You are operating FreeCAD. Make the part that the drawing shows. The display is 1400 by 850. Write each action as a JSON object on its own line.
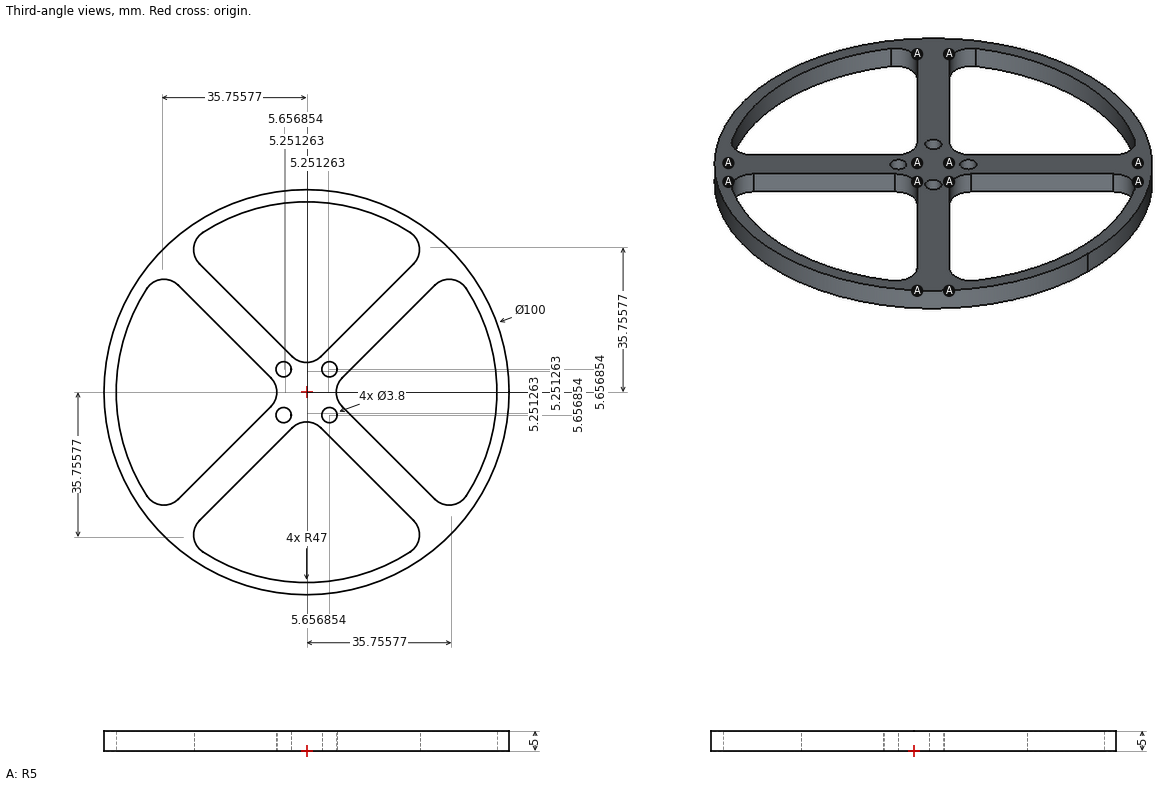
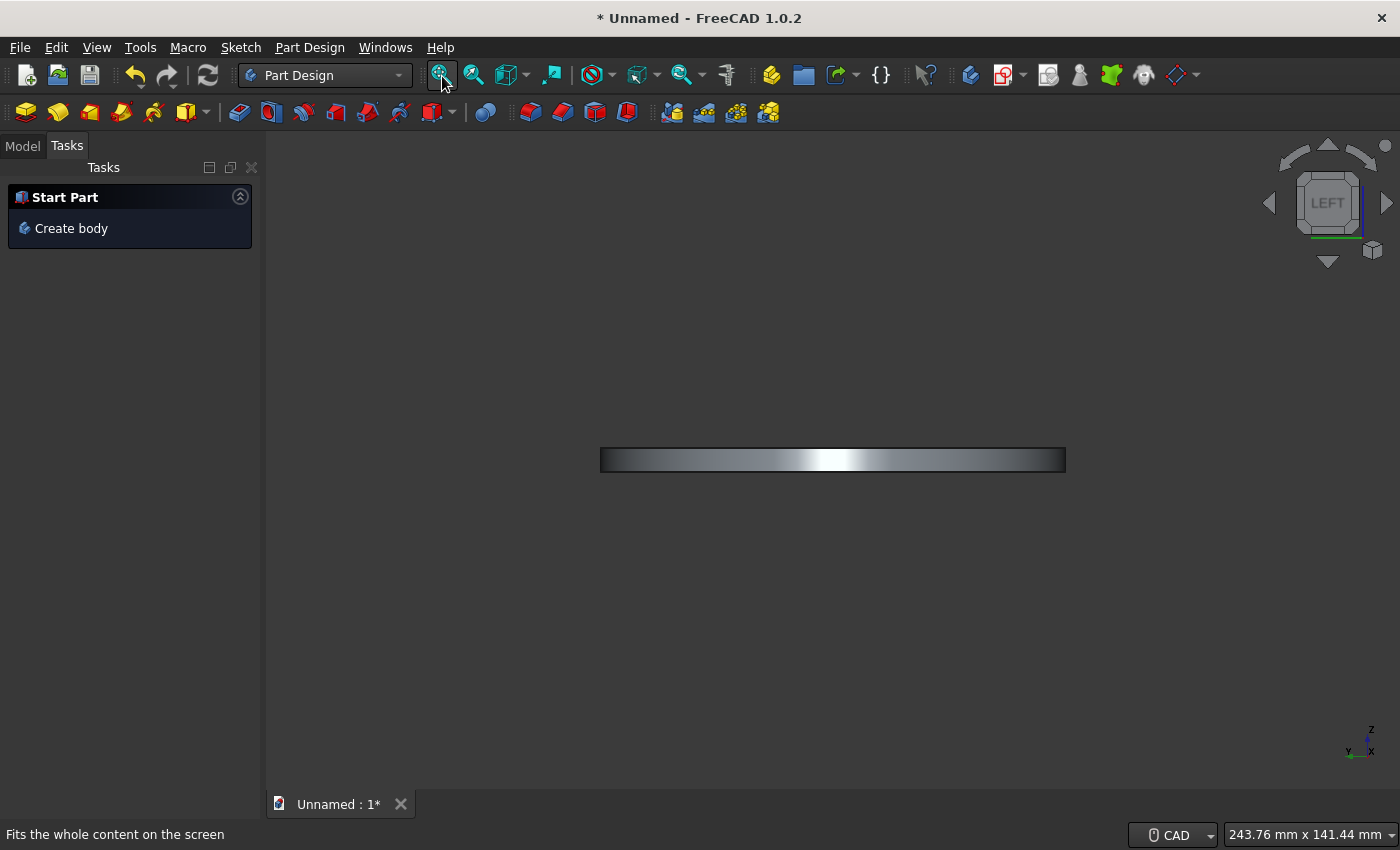
{"action": "key", "text": "v 3"}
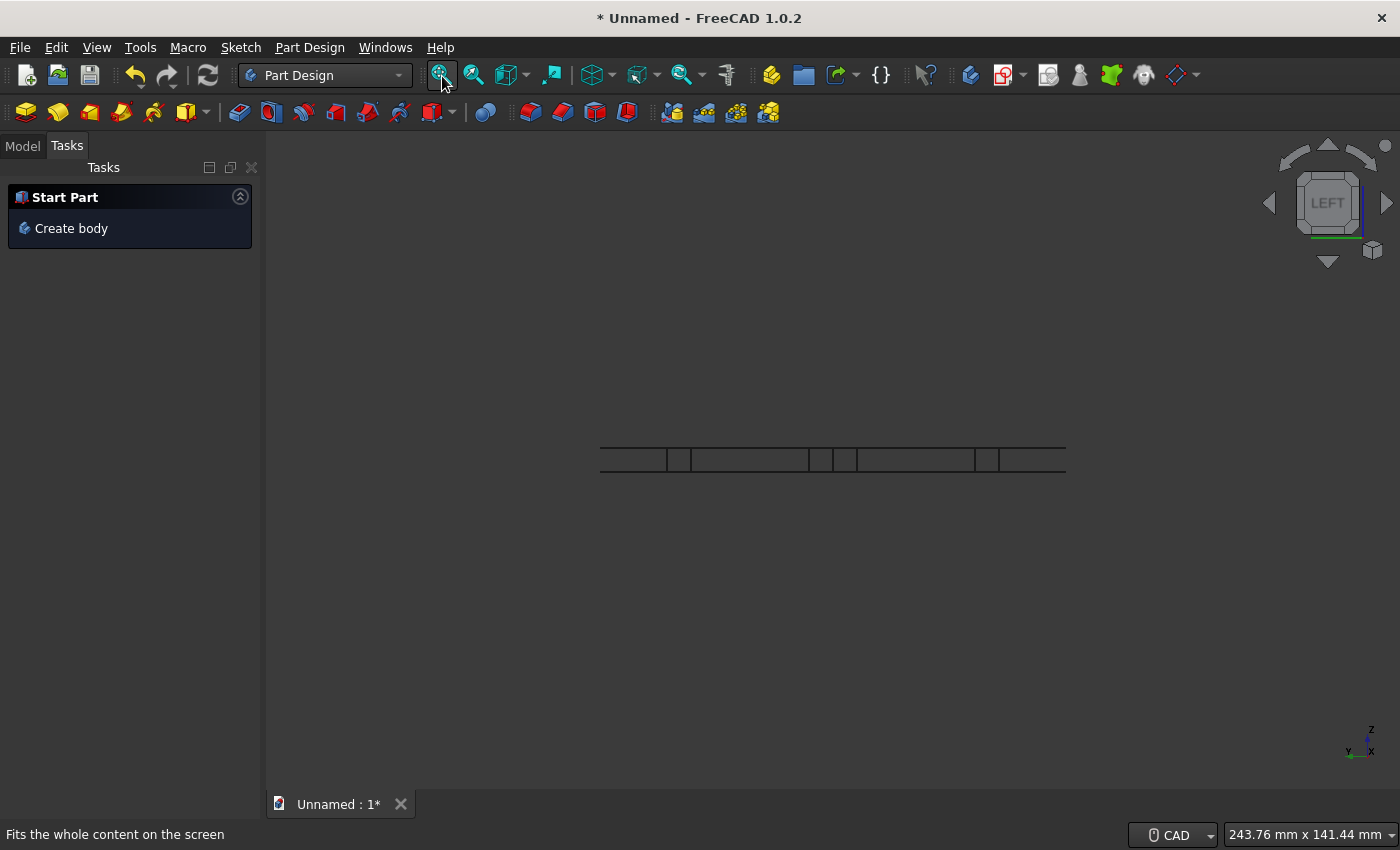
{"action": "key", "text": "0"}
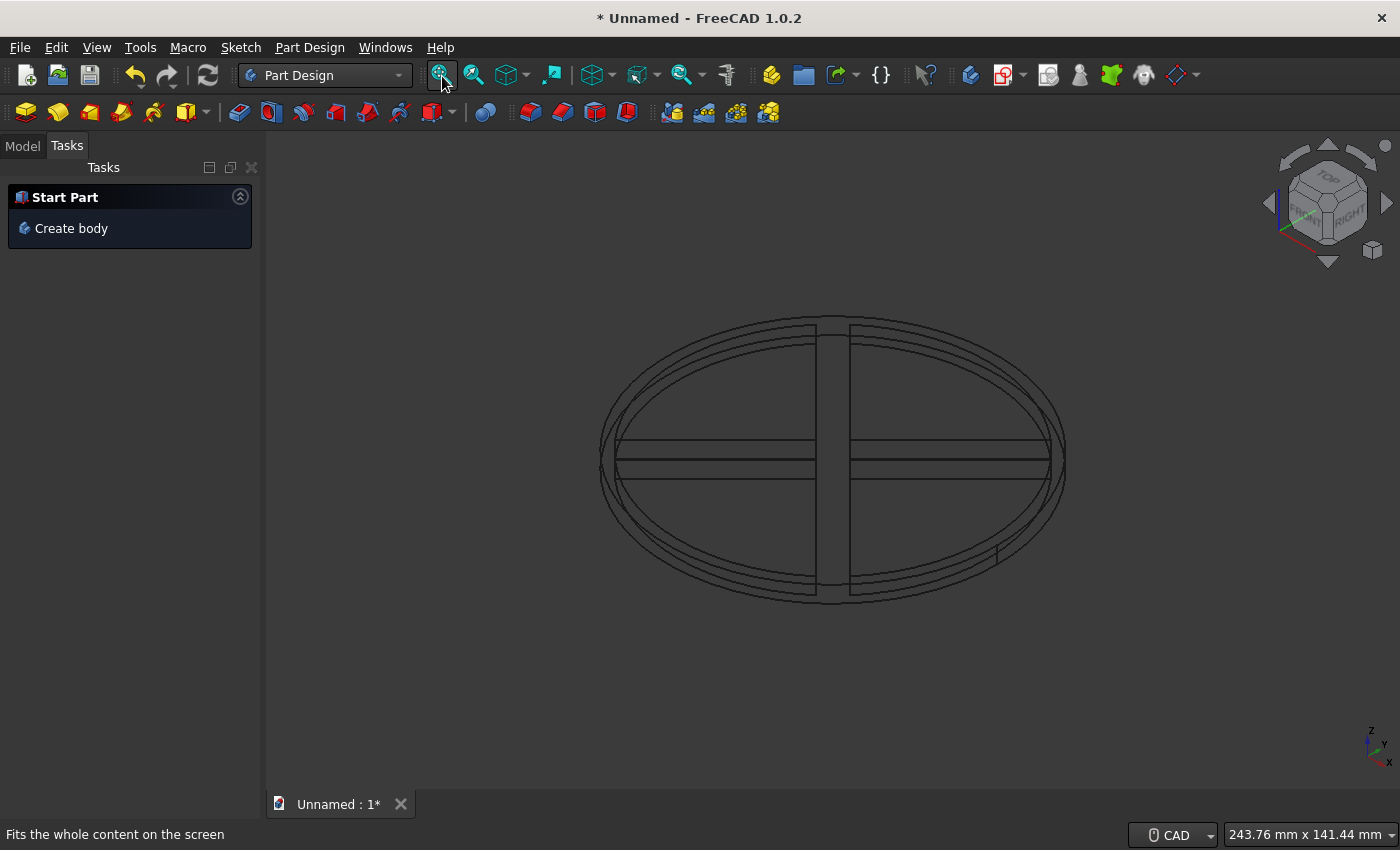
{"action": "left_click", "coordinate": [816, 449]}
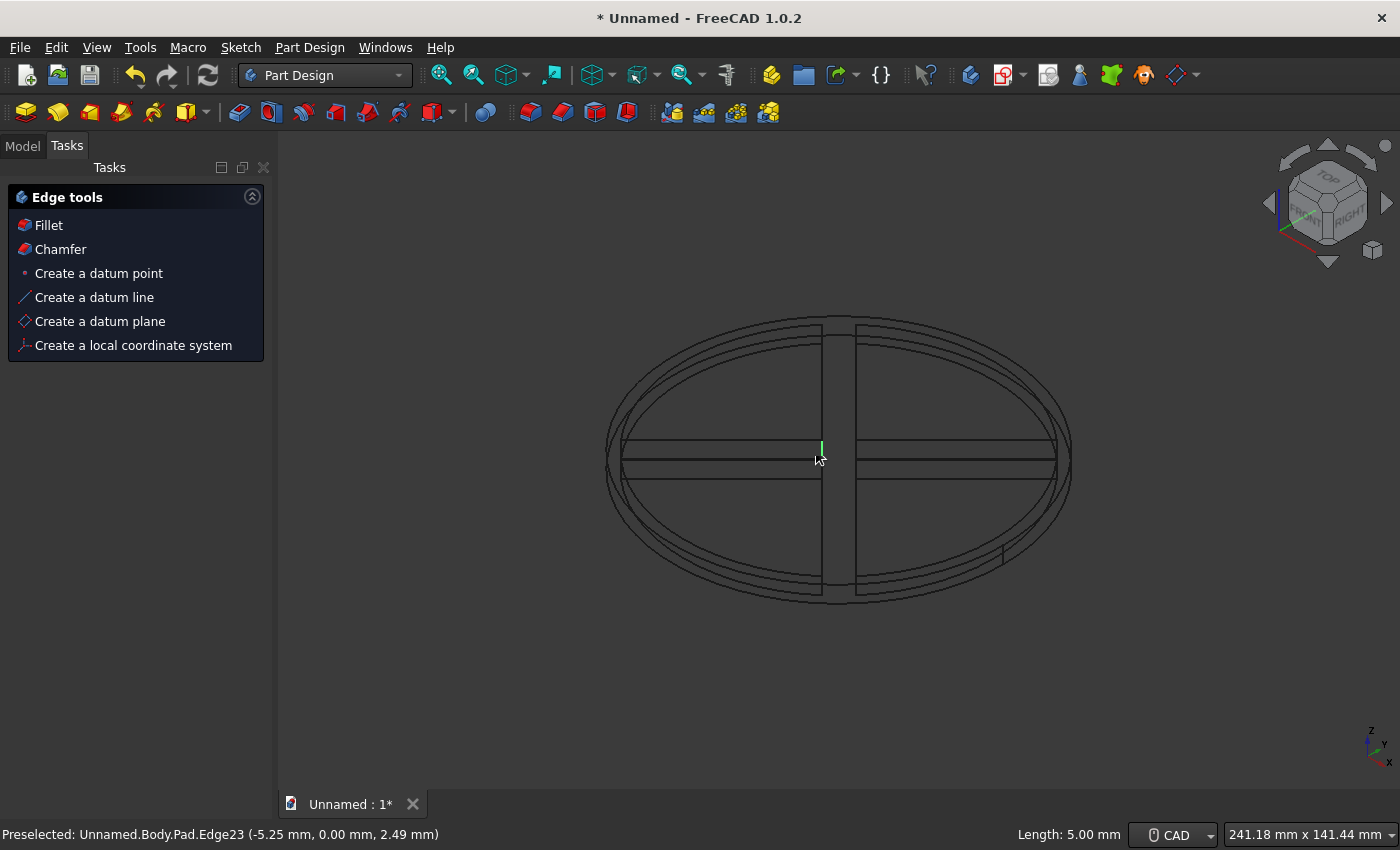
{"action": "left_click", "coordinate": [621, 449], "text": "ctrl"}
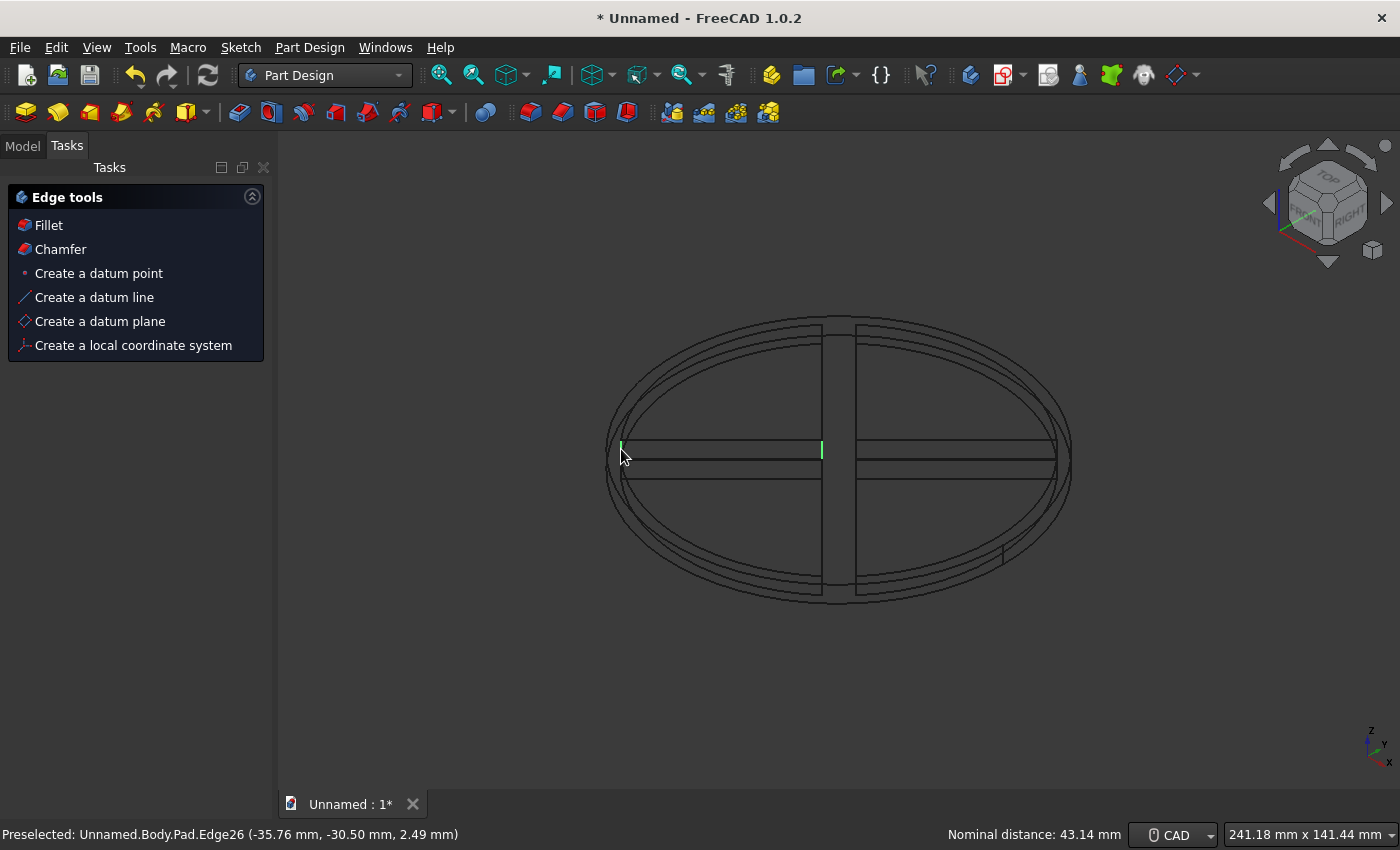
{"action": "left_click", "coordinate": [856, 590], "text": "ctrl"}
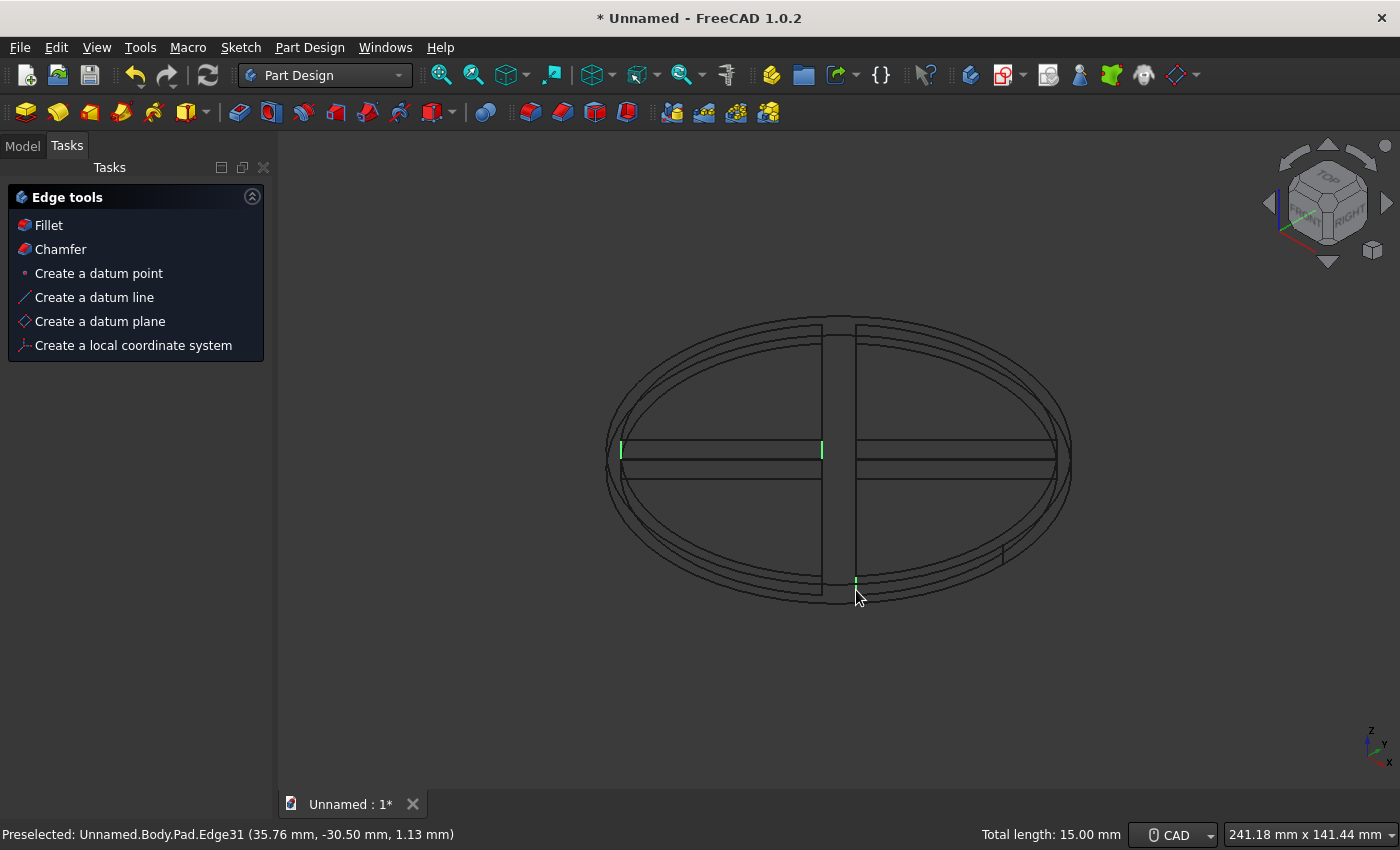
{"action": "left_click", "coordinate": [822, 590], "text": "ctrl"}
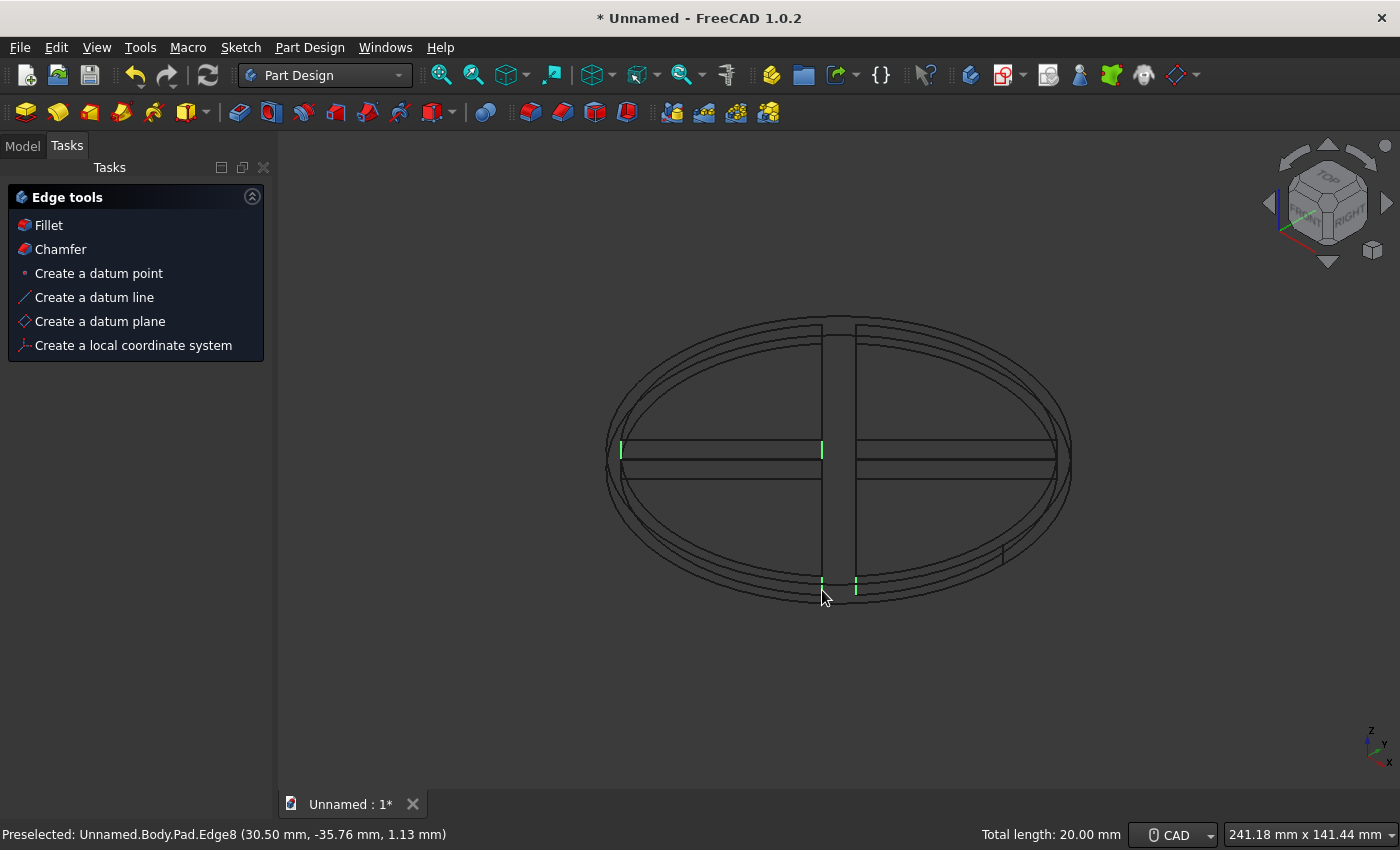
{"action": "left_click", "coordinate": [1057, 449], "text": "ctrl"}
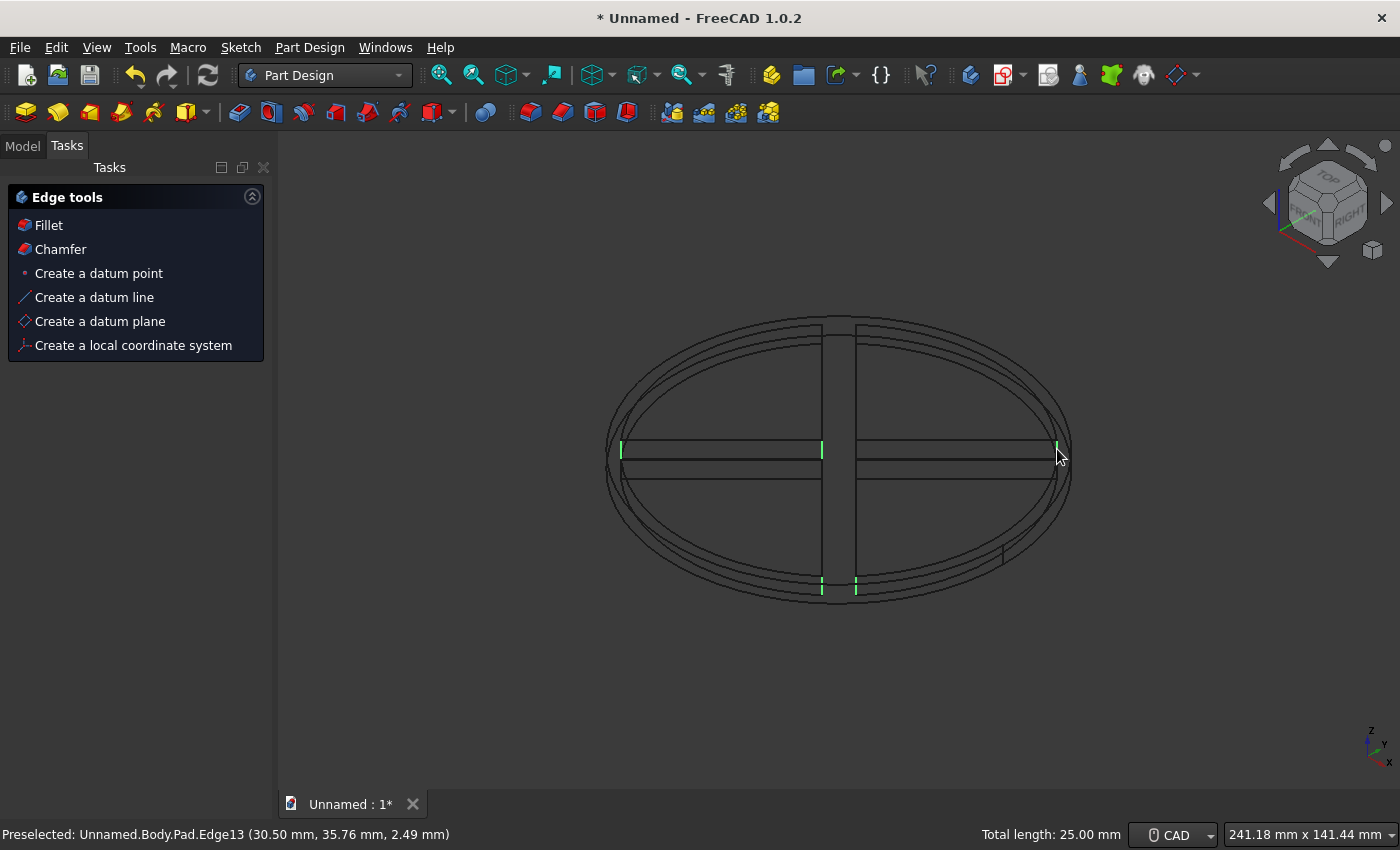
{"action": "left_click", "coordinate": [856, 449], "text": "ctrl"}